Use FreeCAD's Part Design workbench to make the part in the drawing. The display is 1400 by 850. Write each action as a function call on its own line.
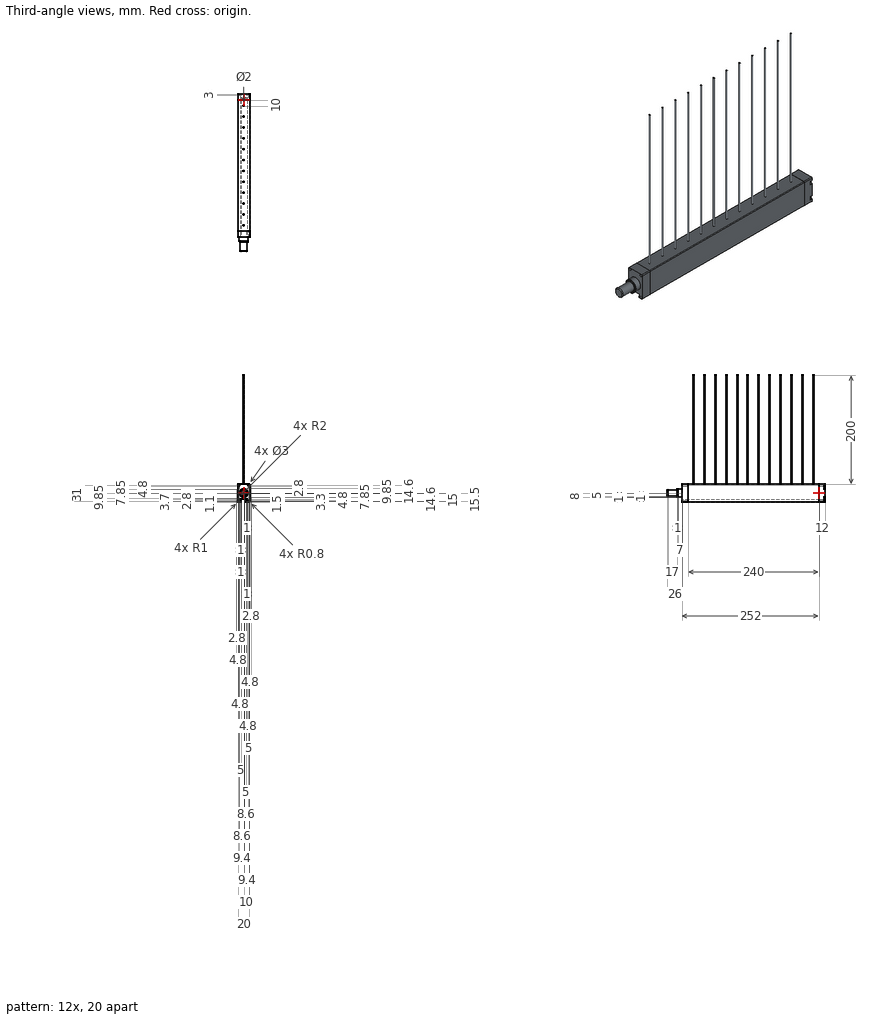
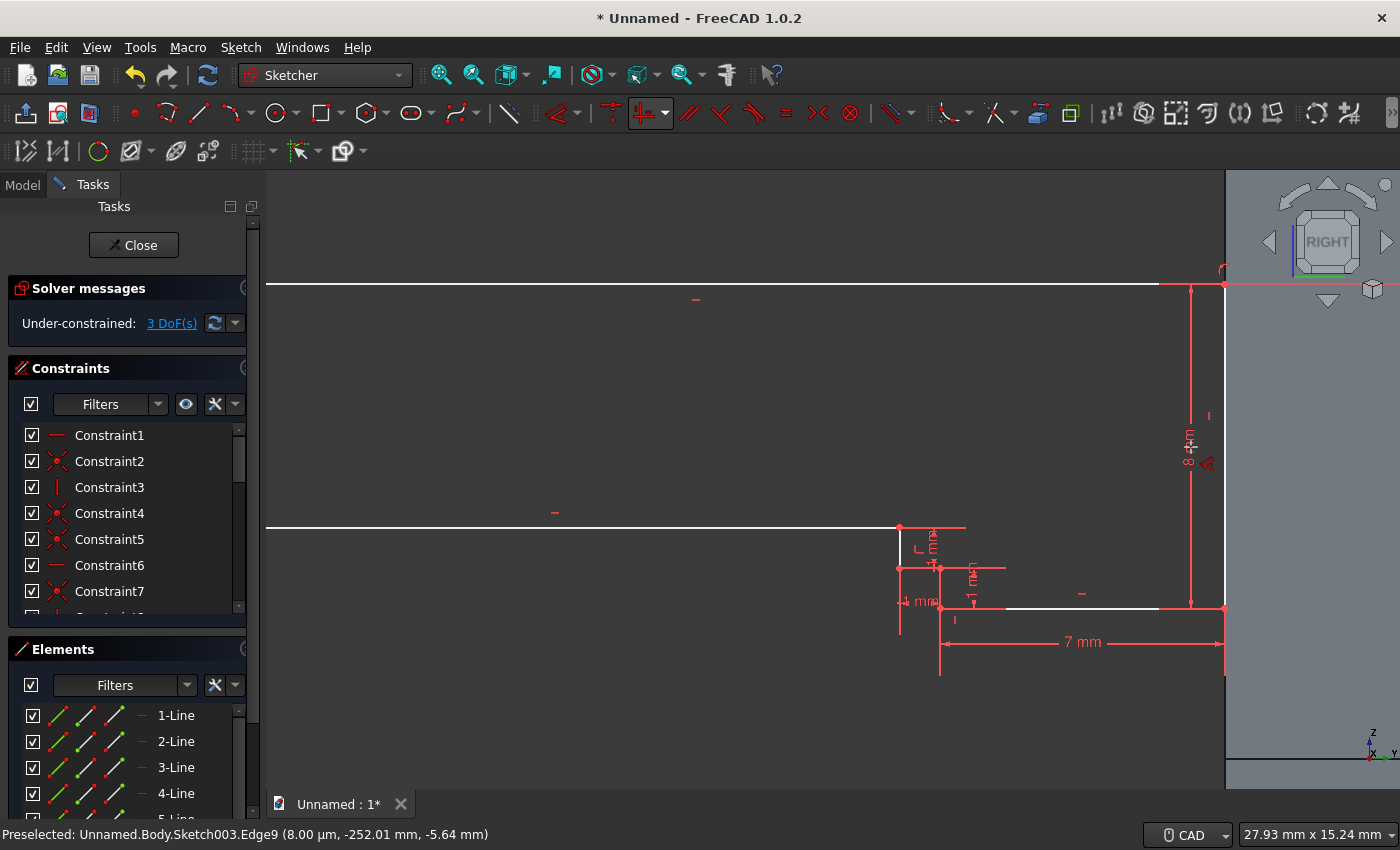
click(908, 284)
click(759, 250)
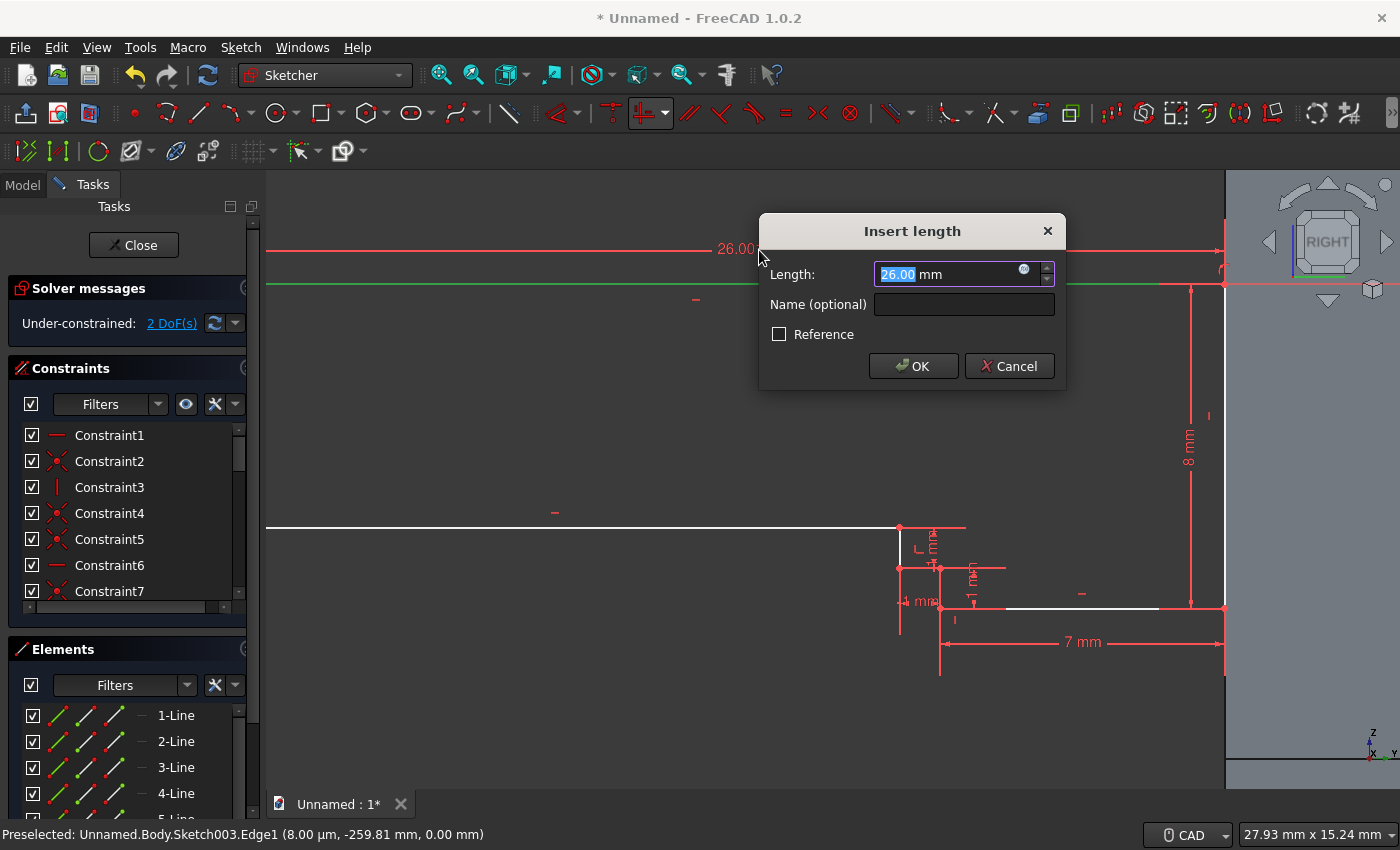
text(26)
key(Return)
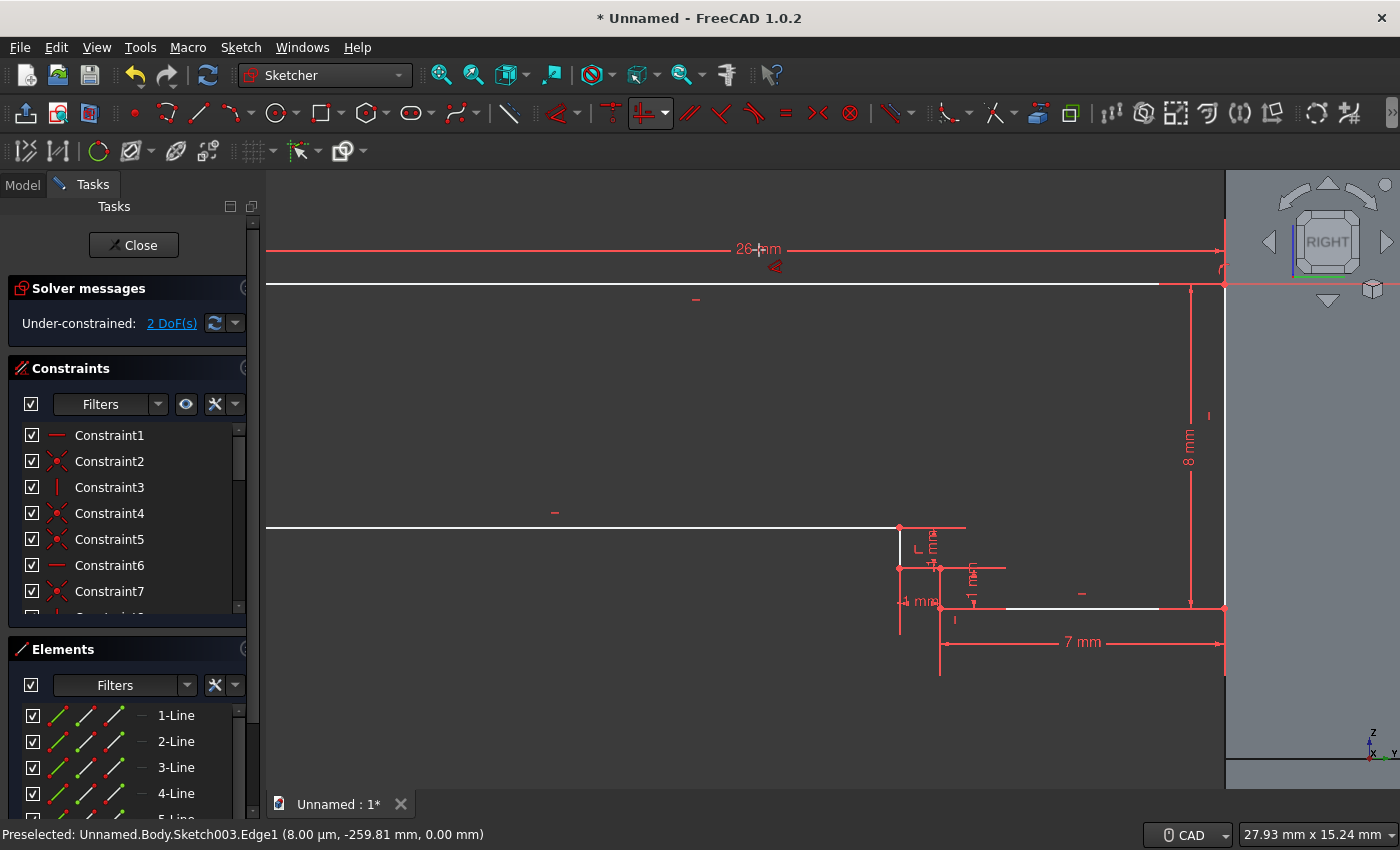
click(417, 528)
click(597, 562)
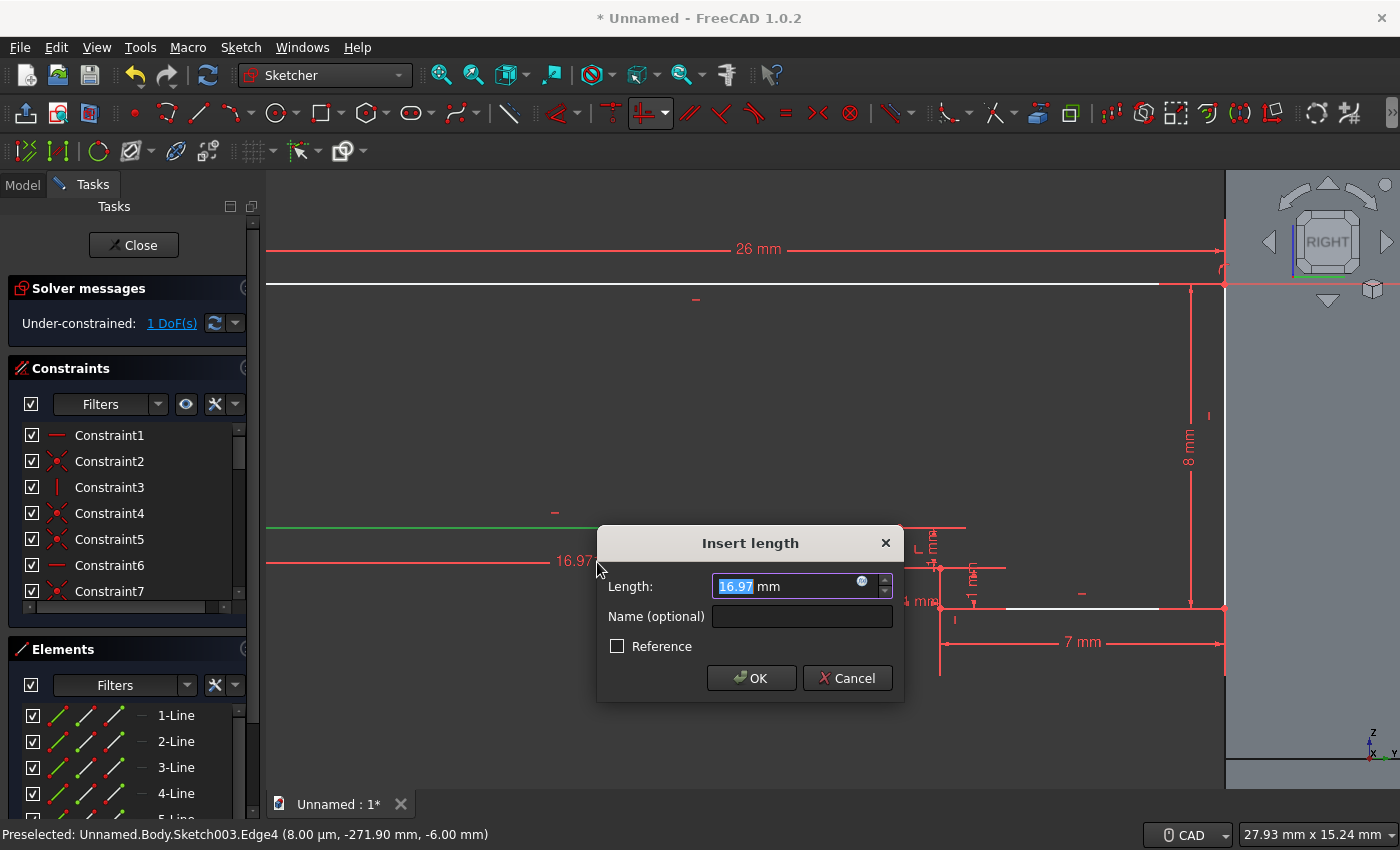
text(17)
key(Return)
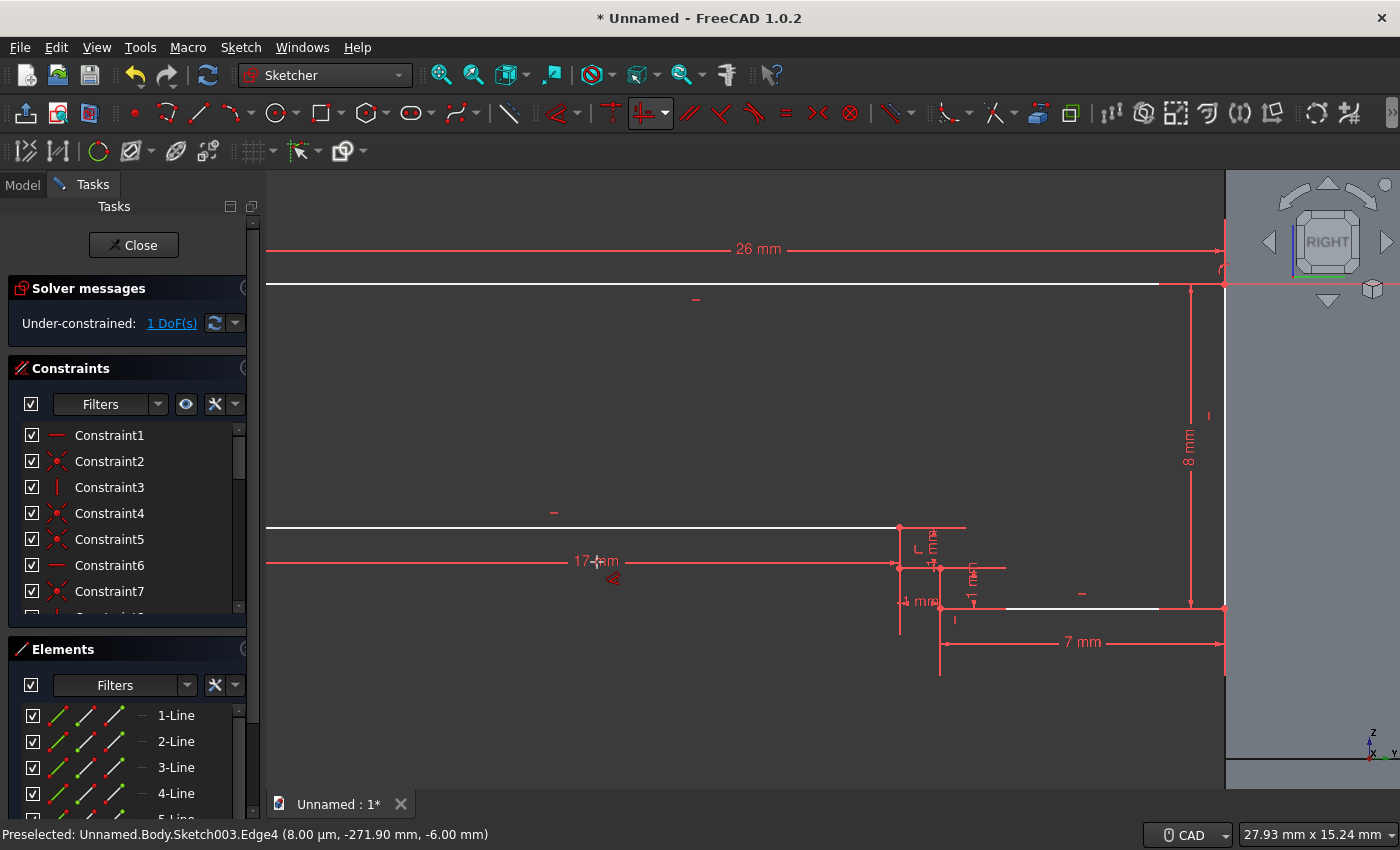
click(1225, 284)
click(1230, 250)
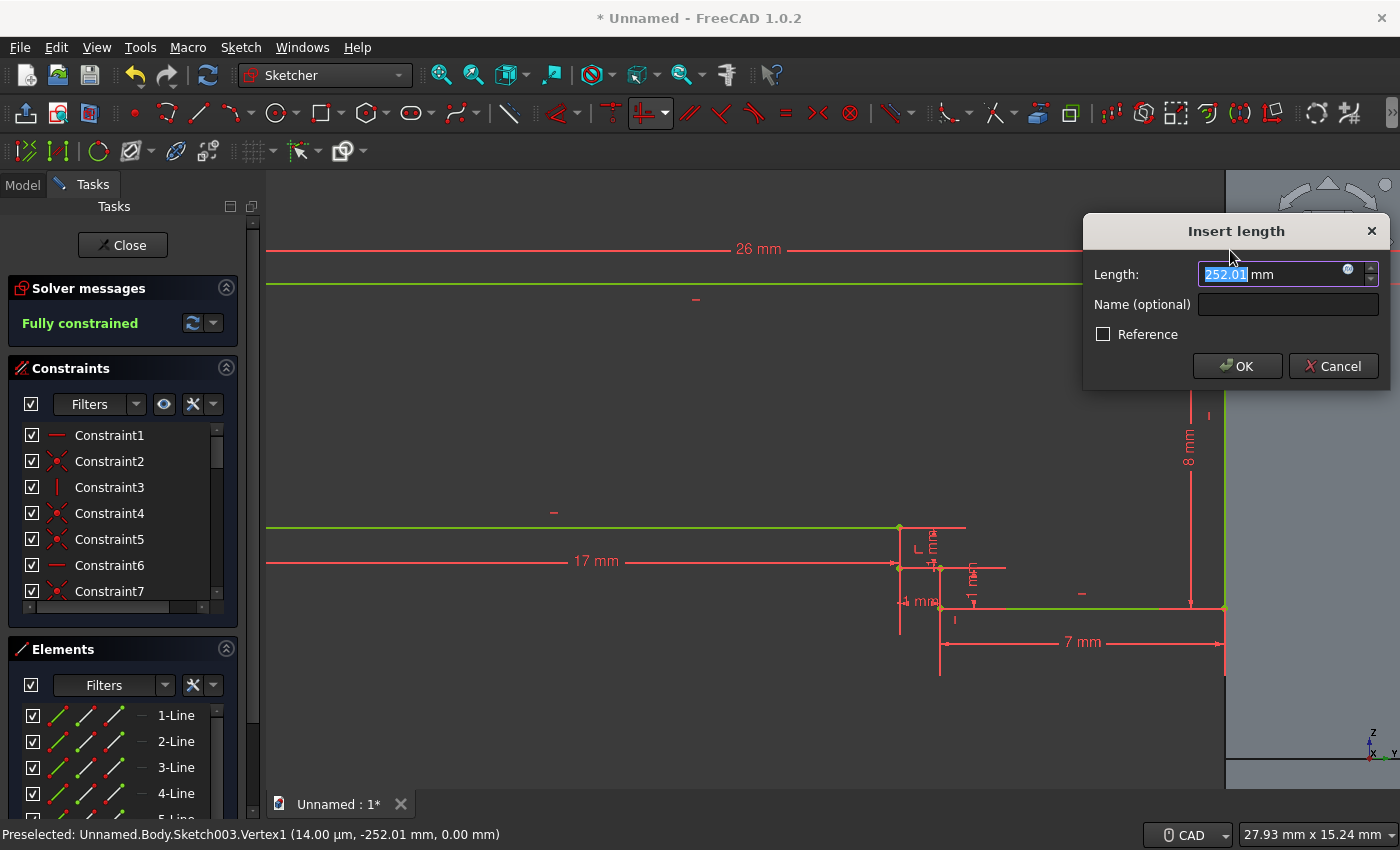
text(252)
key(Return)
key(Escape)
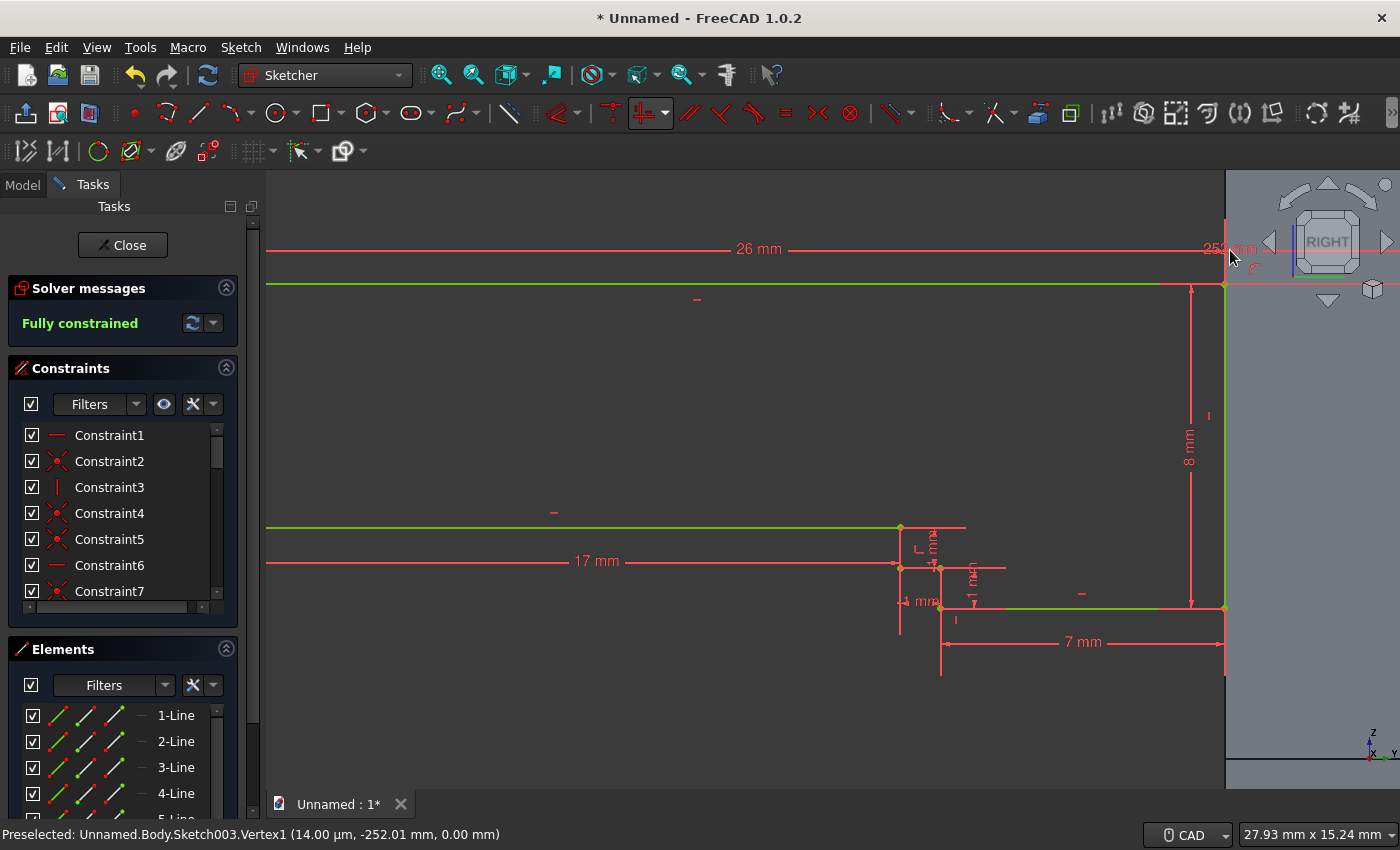
click(123, 245)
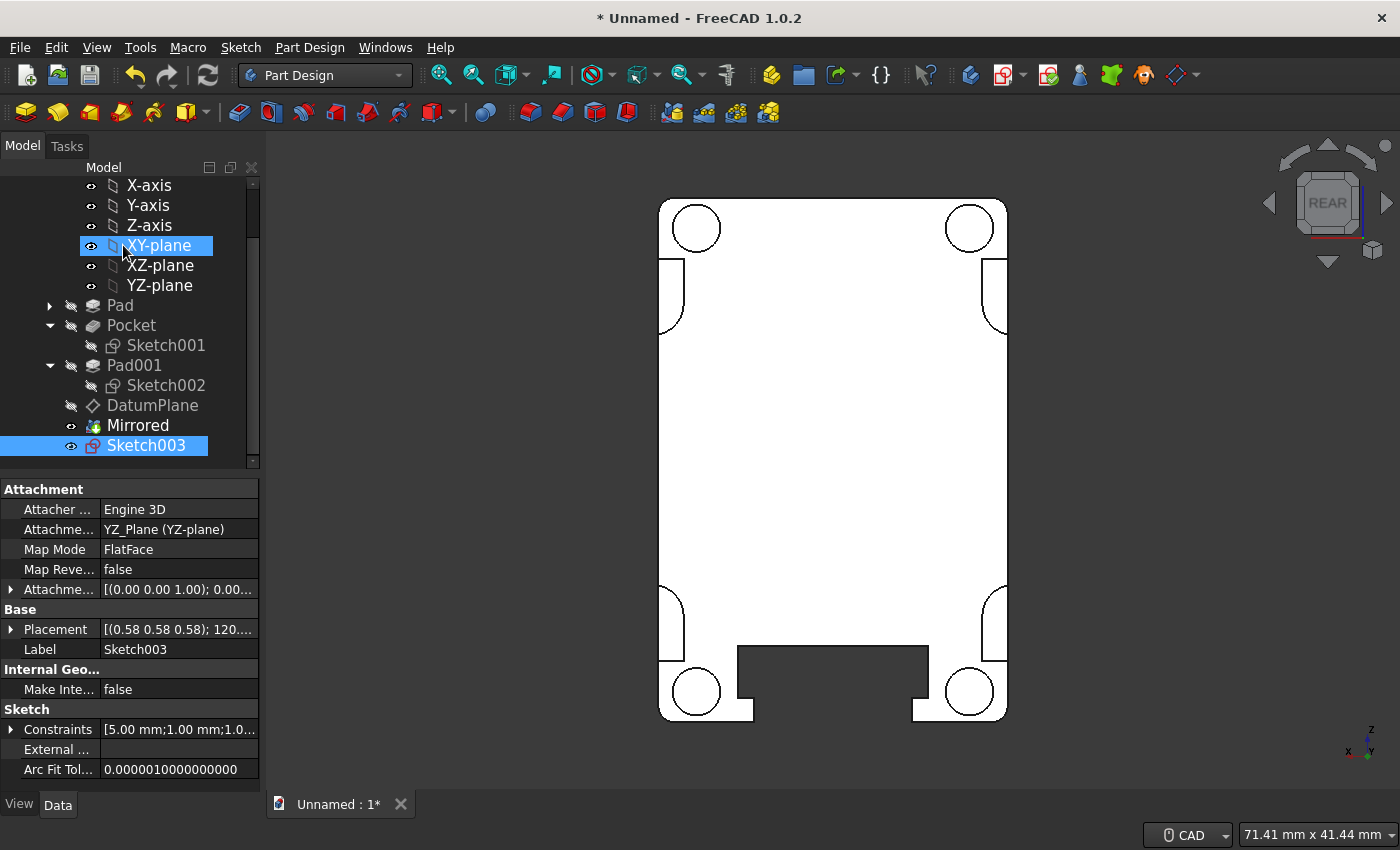
click(58, 112)